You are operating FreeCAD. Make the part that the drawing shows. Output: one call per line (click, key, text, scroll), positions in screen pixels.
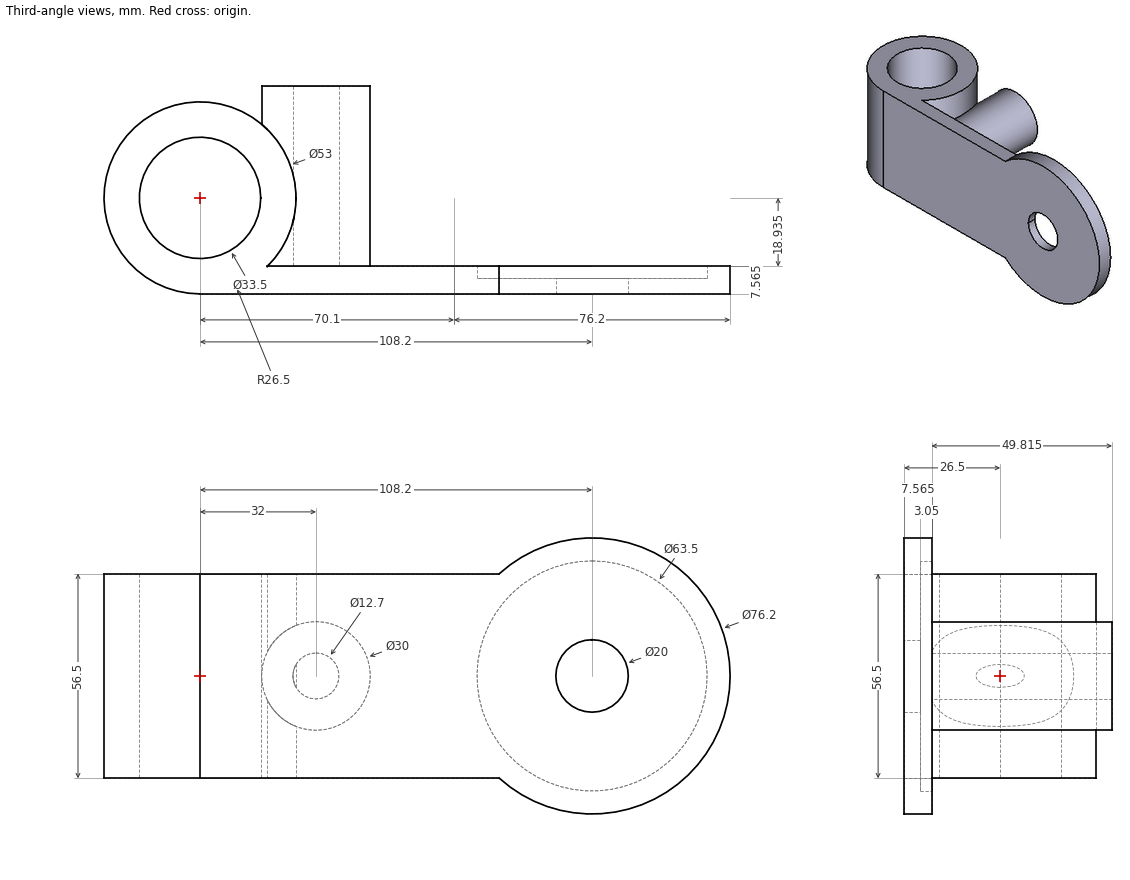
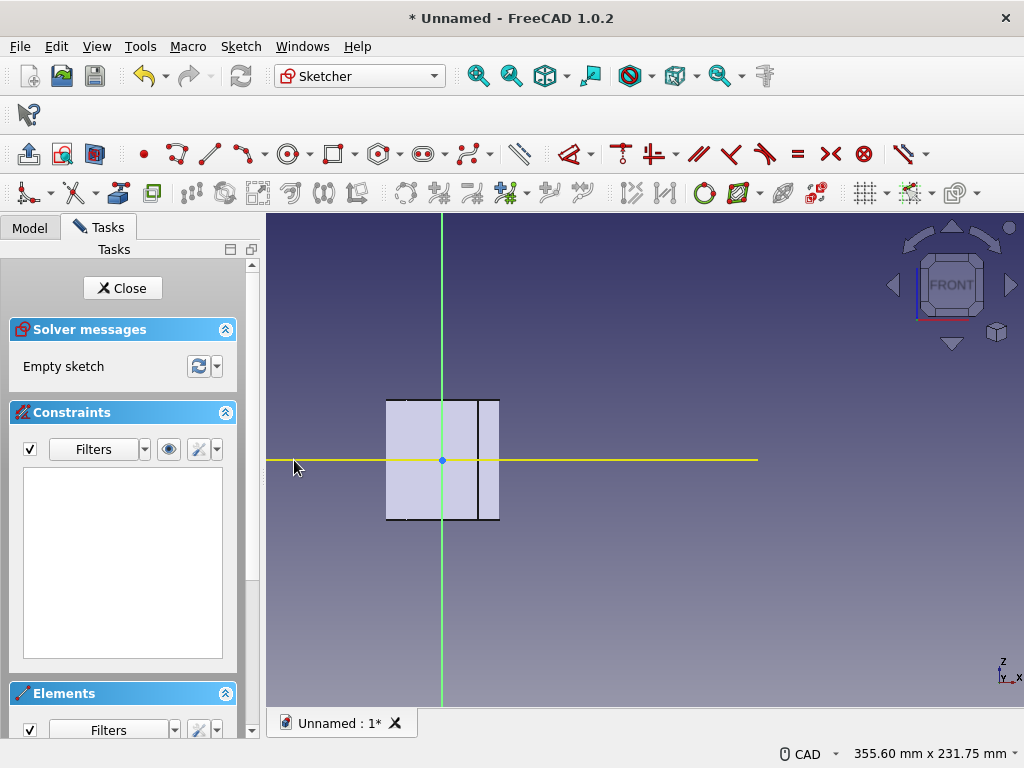
key(g)
key(c)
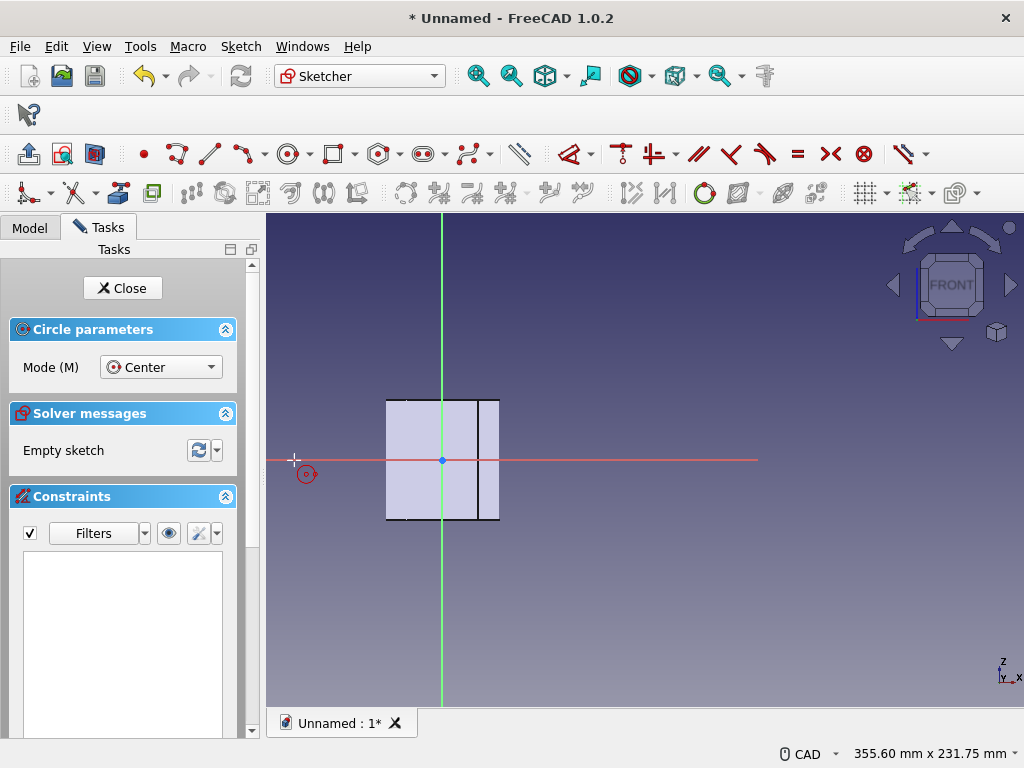
click(673, 460)
move(730, 403)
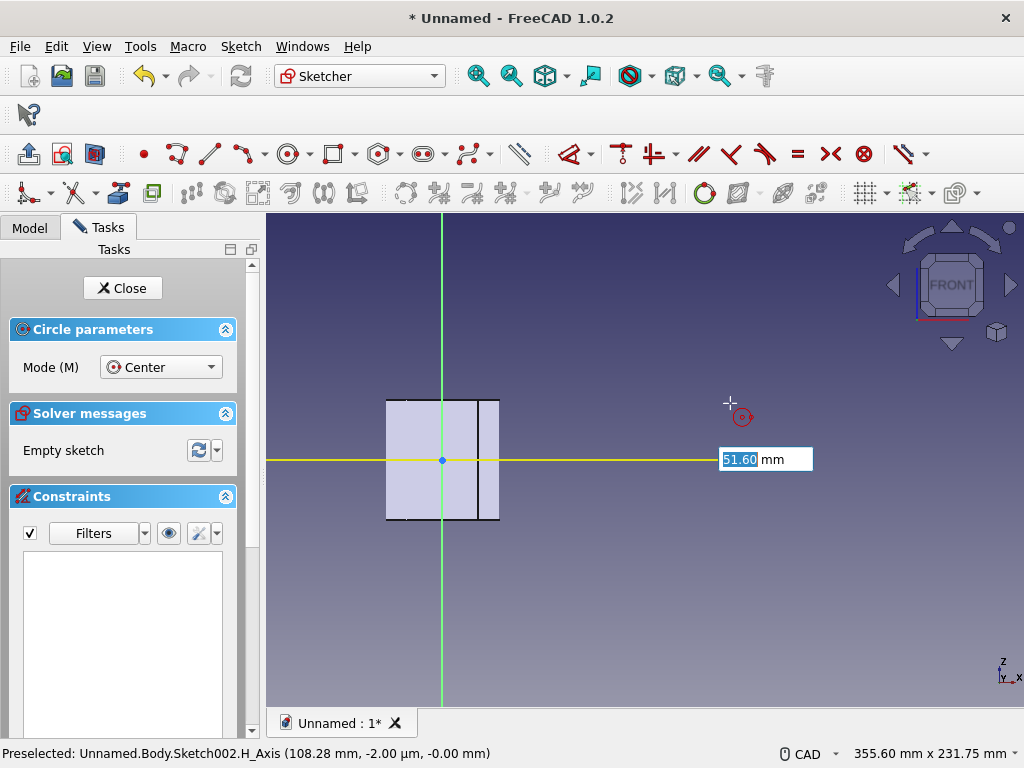
text(76.2)
key(Return)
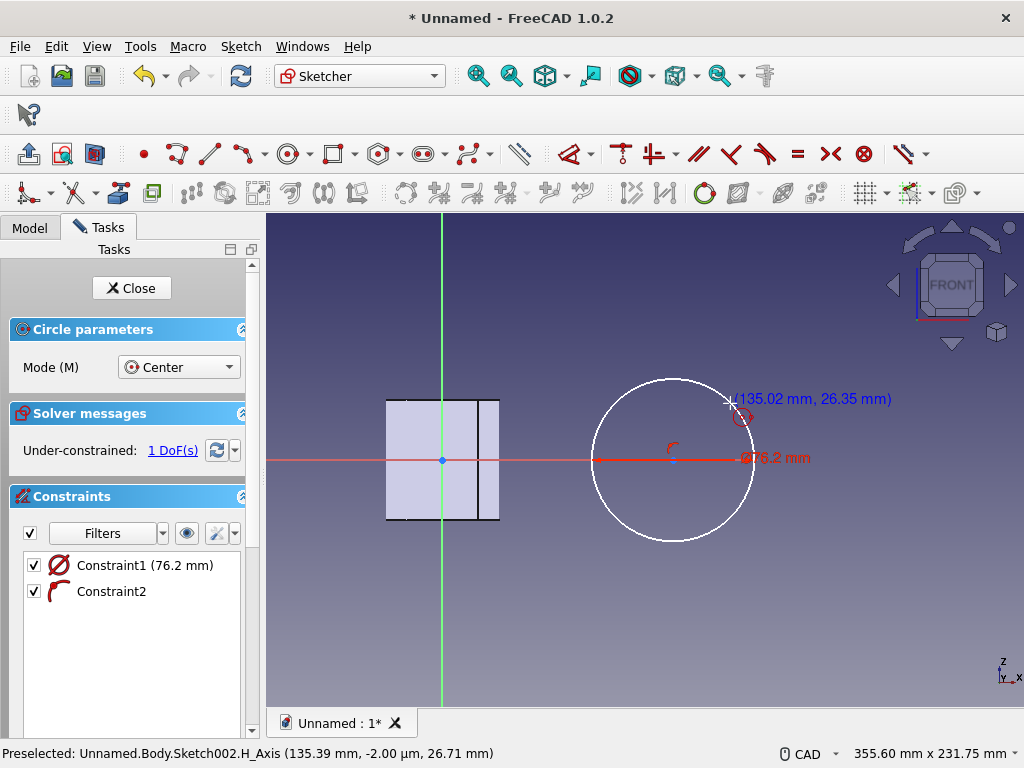
click(673, 460)
move(721, 412)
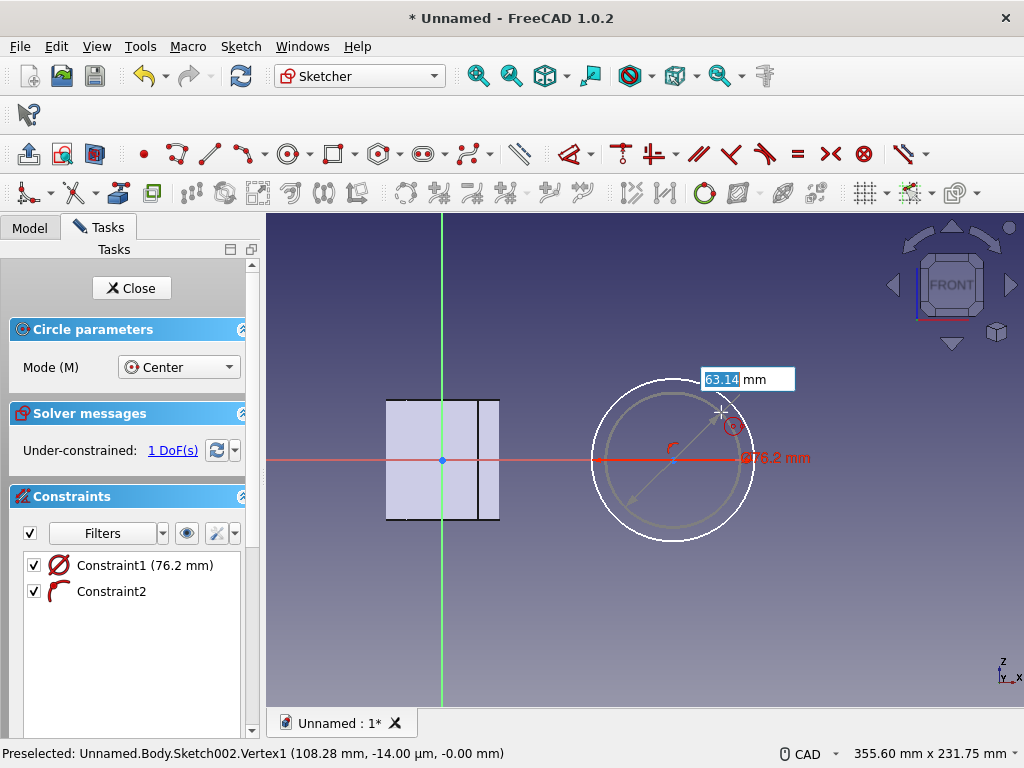
text(63.5)
key(Return)
key(Escape)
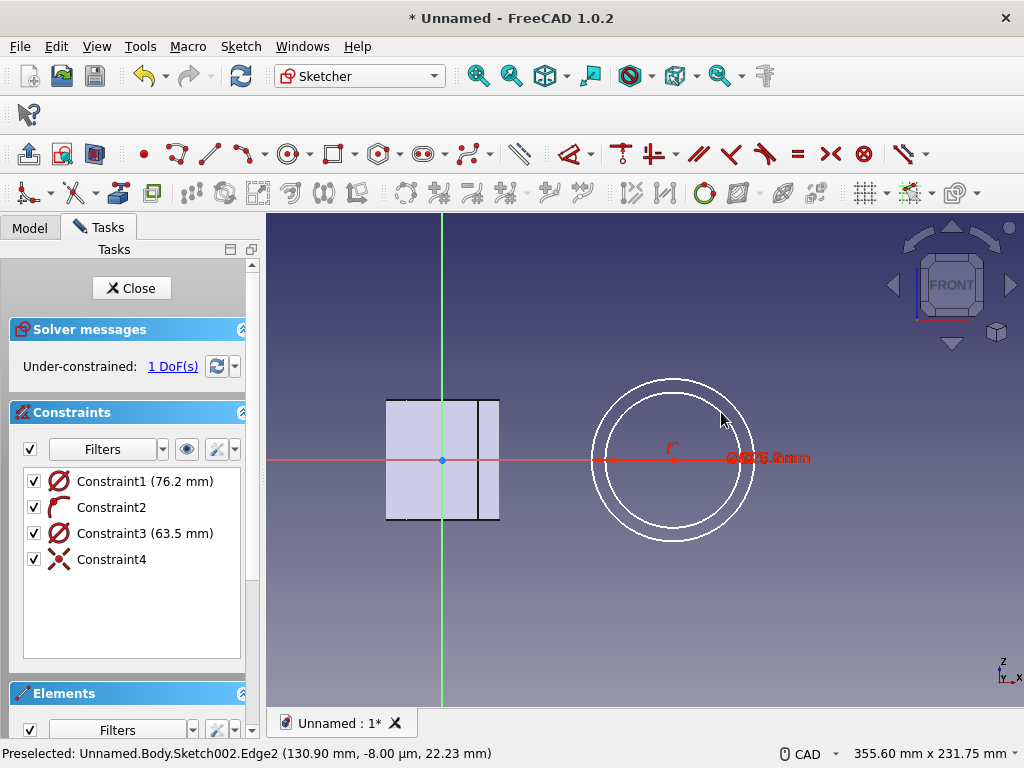
key(d)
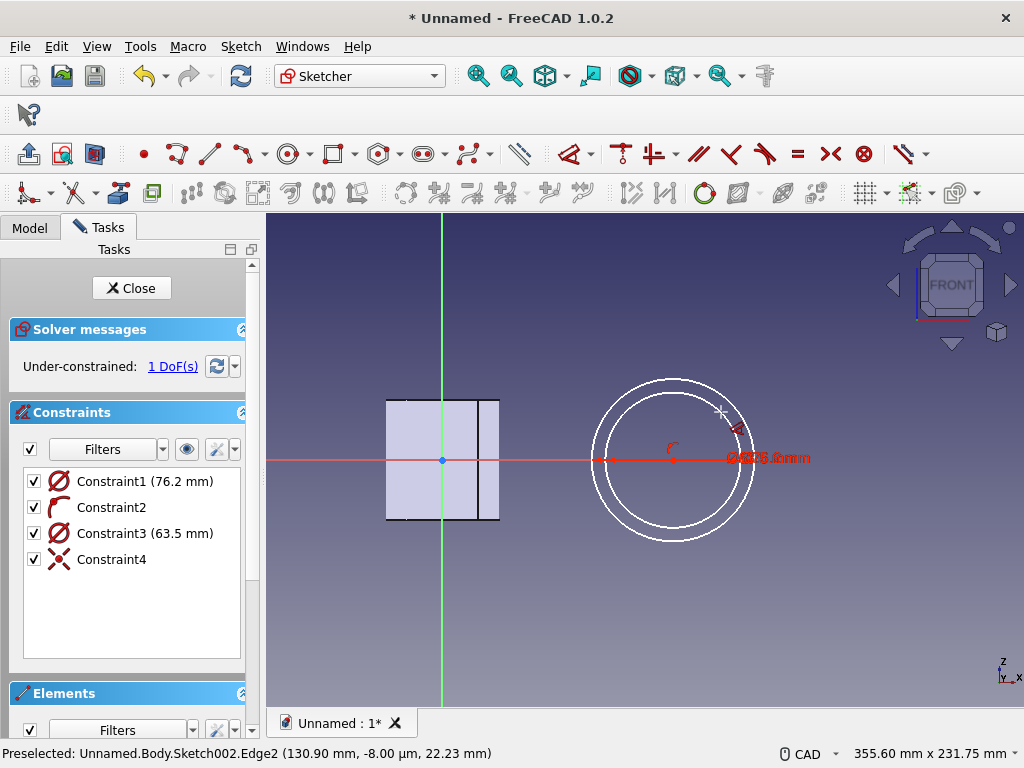
click(673, 460)
click(558, 494)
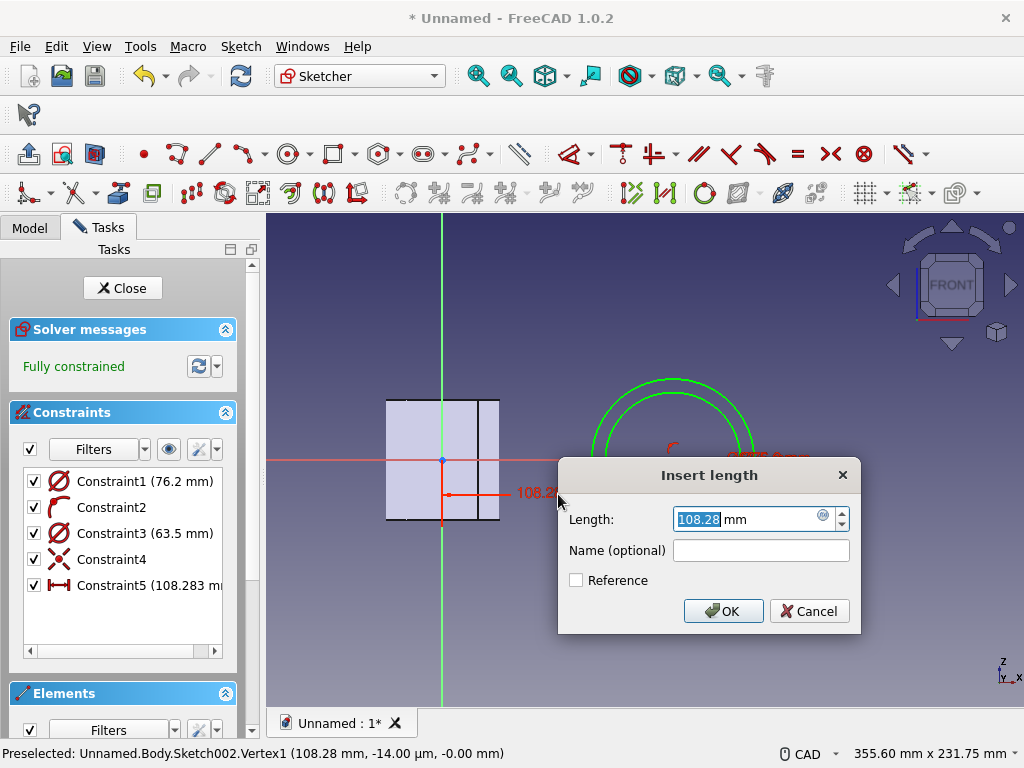
text(108.2)
key(Return)
key(Escape)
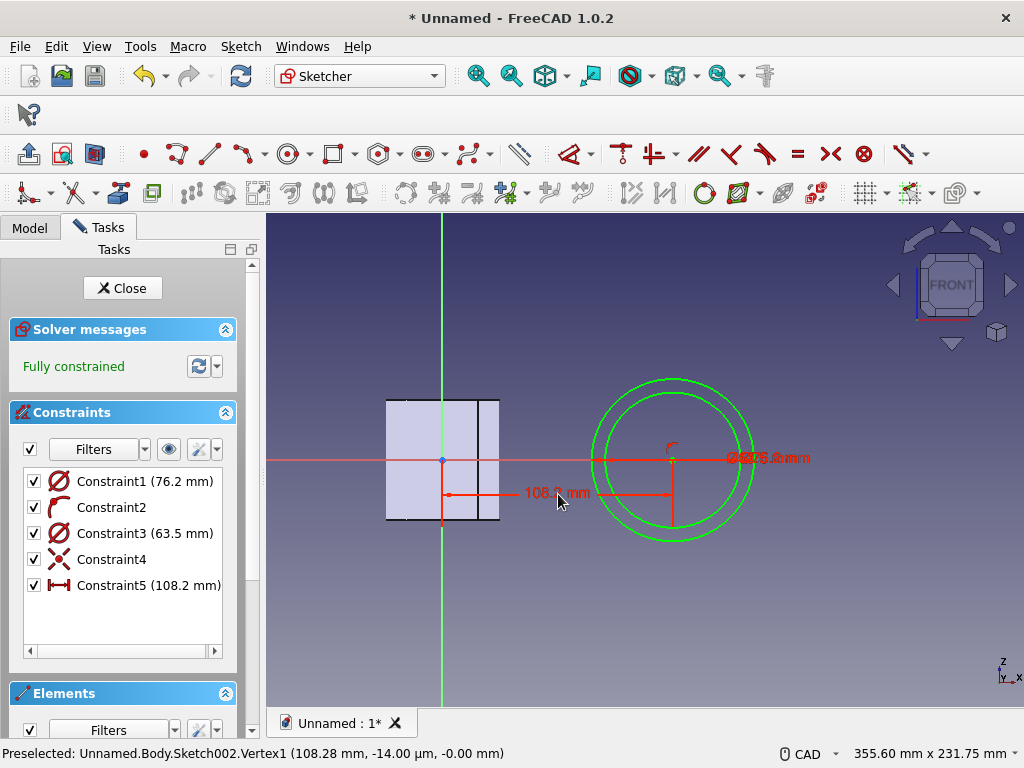
click(123, 288)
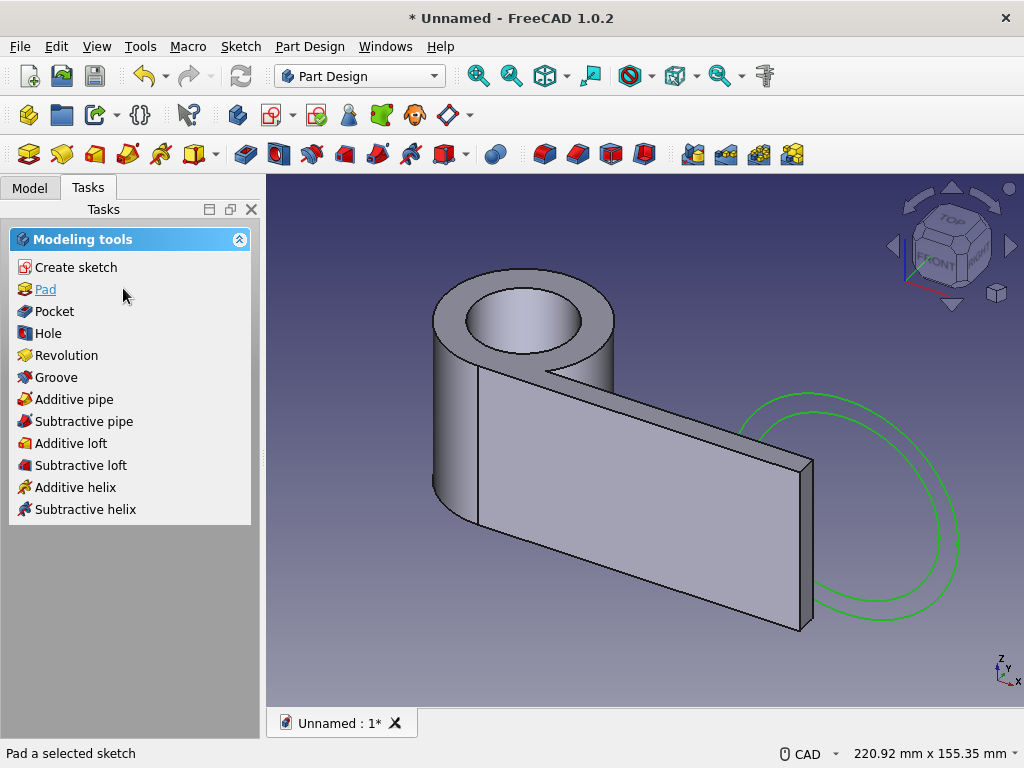
click(29, 154)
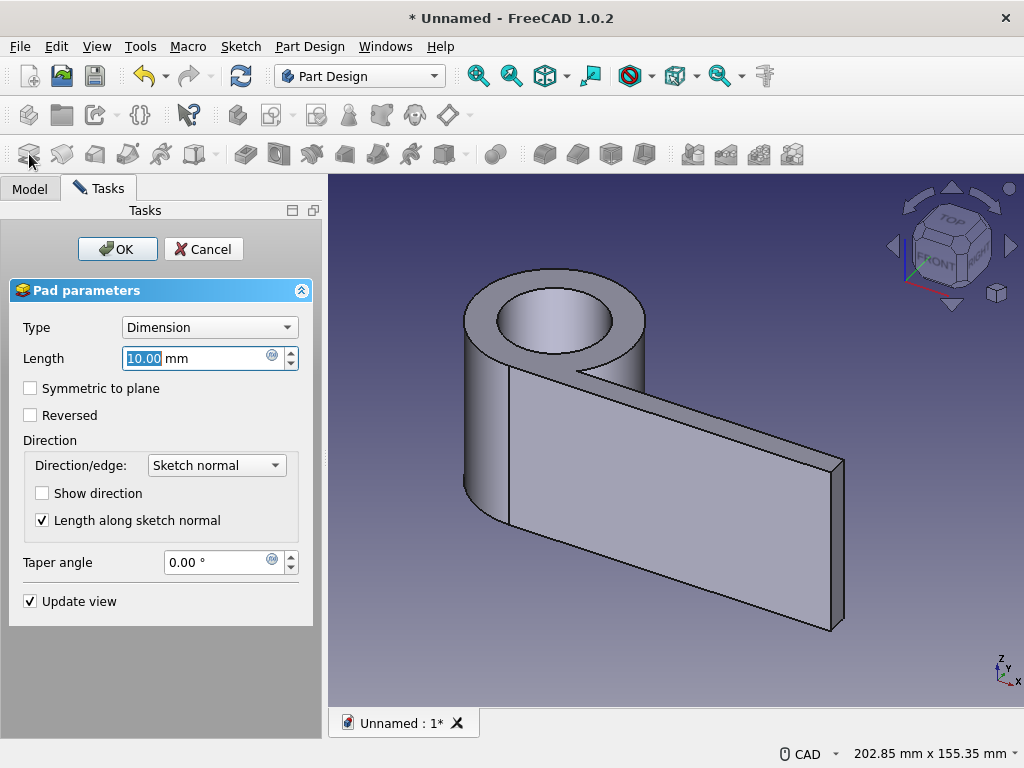
text(26.5)
key(Tab)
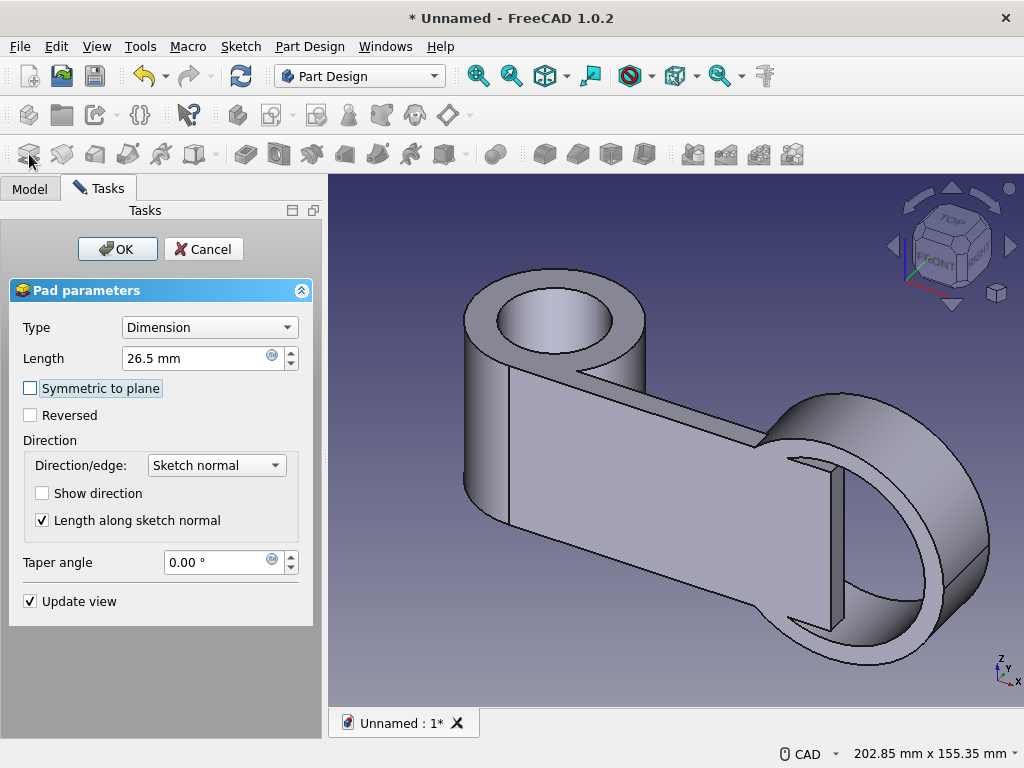
click(118, 249)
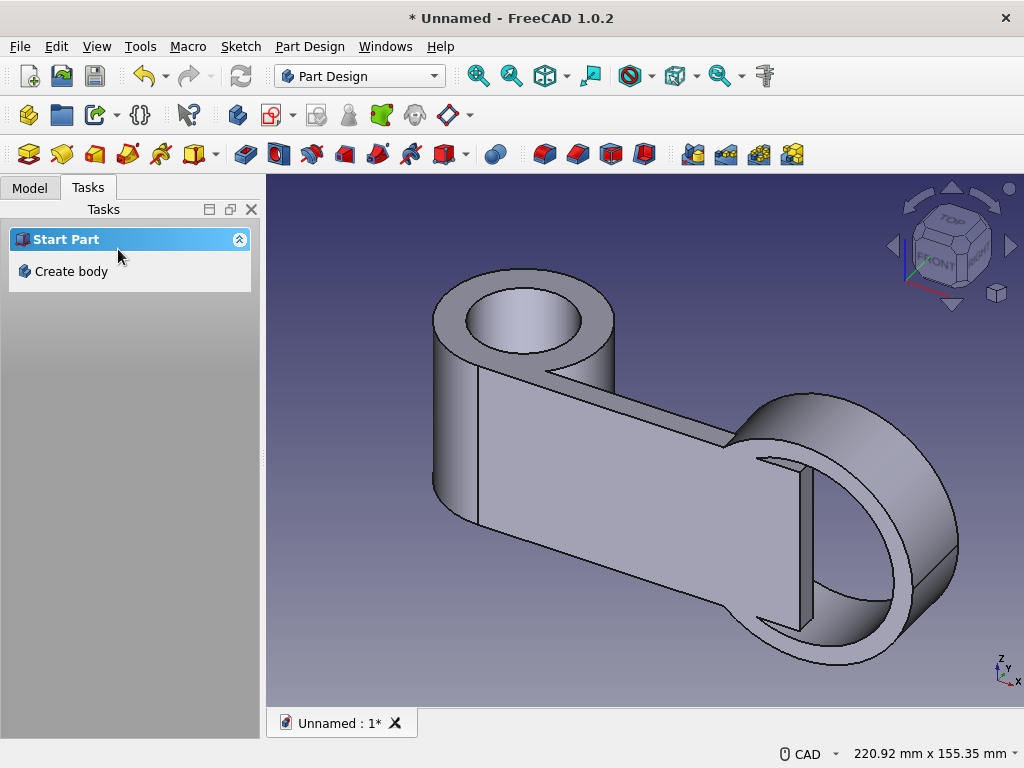
click(270, 116)